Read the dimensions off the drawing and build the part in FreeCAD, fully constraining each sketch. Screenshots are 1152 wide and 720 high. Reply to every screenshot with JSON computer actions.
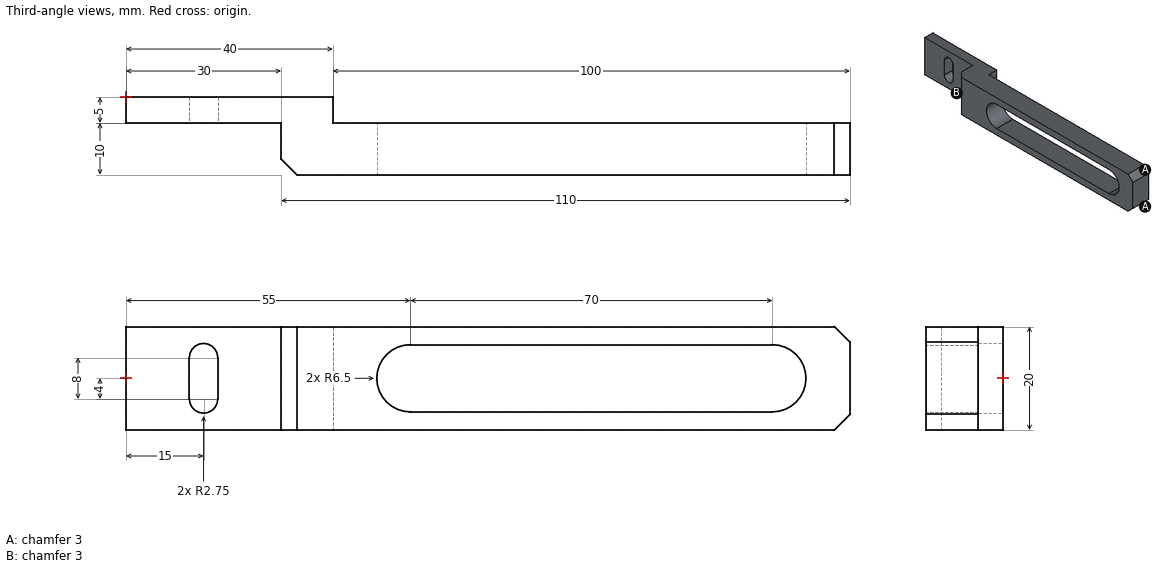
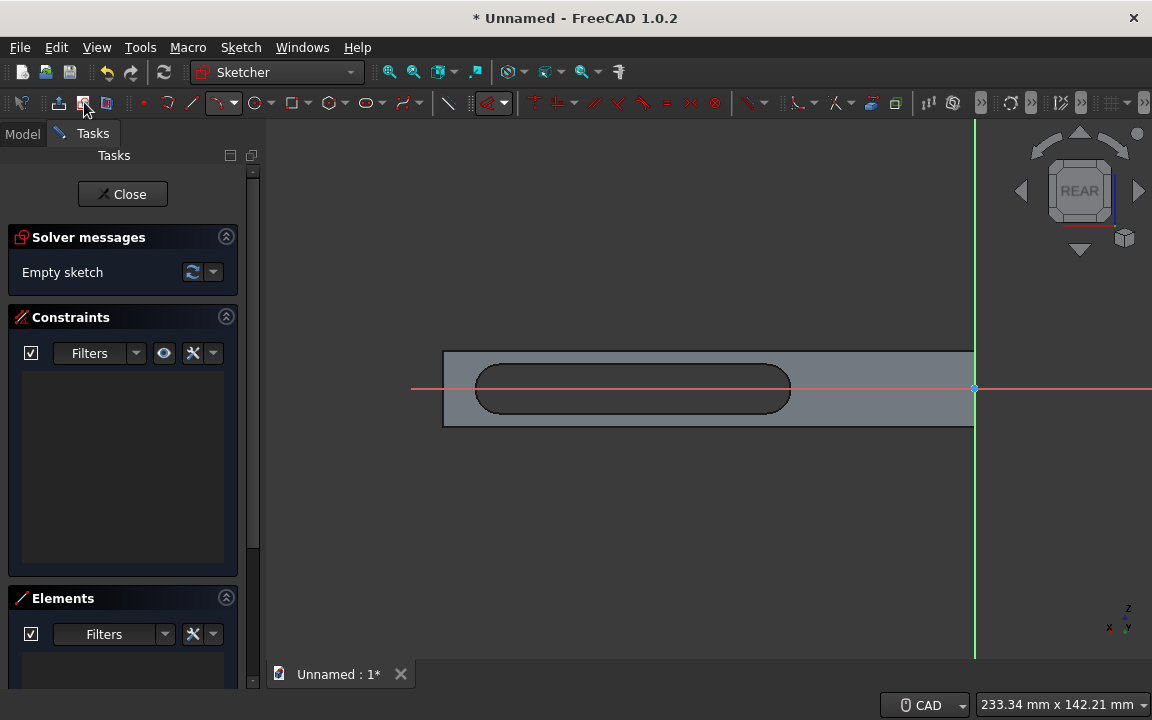
{"action": "scroll", "coordinate": [987, 389], "scroll_direction": "up", "scroll_amount": 9}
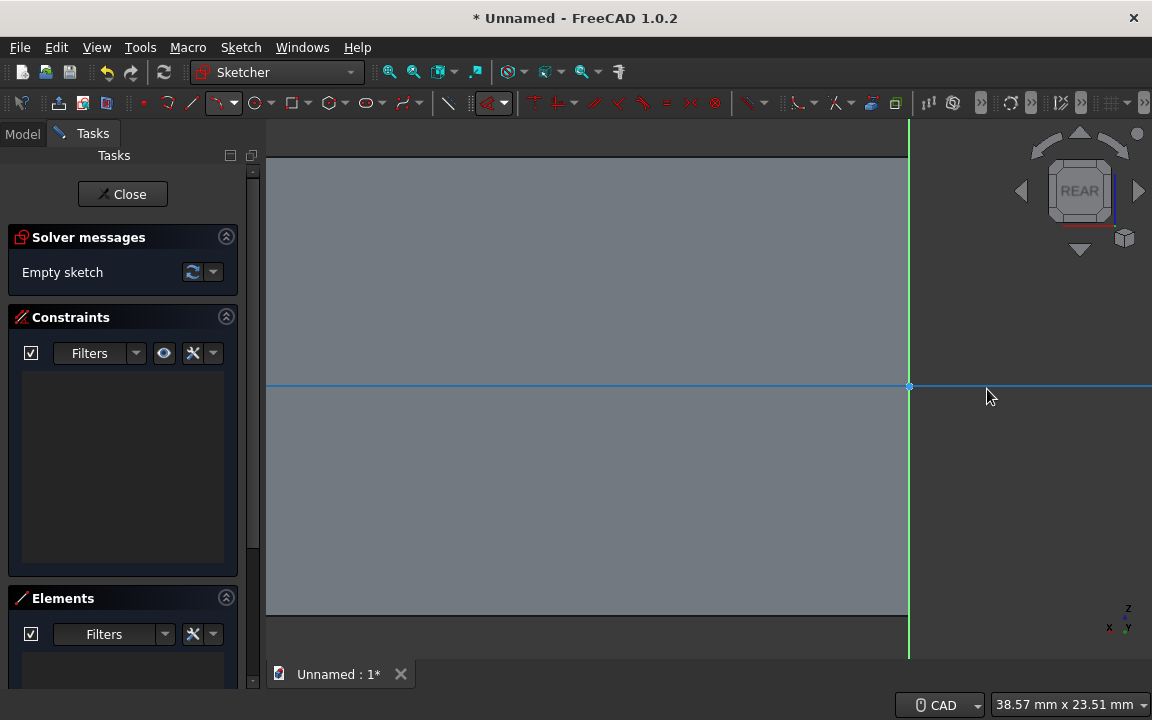
{"action": "left_click", "coordinate": [366, 104]}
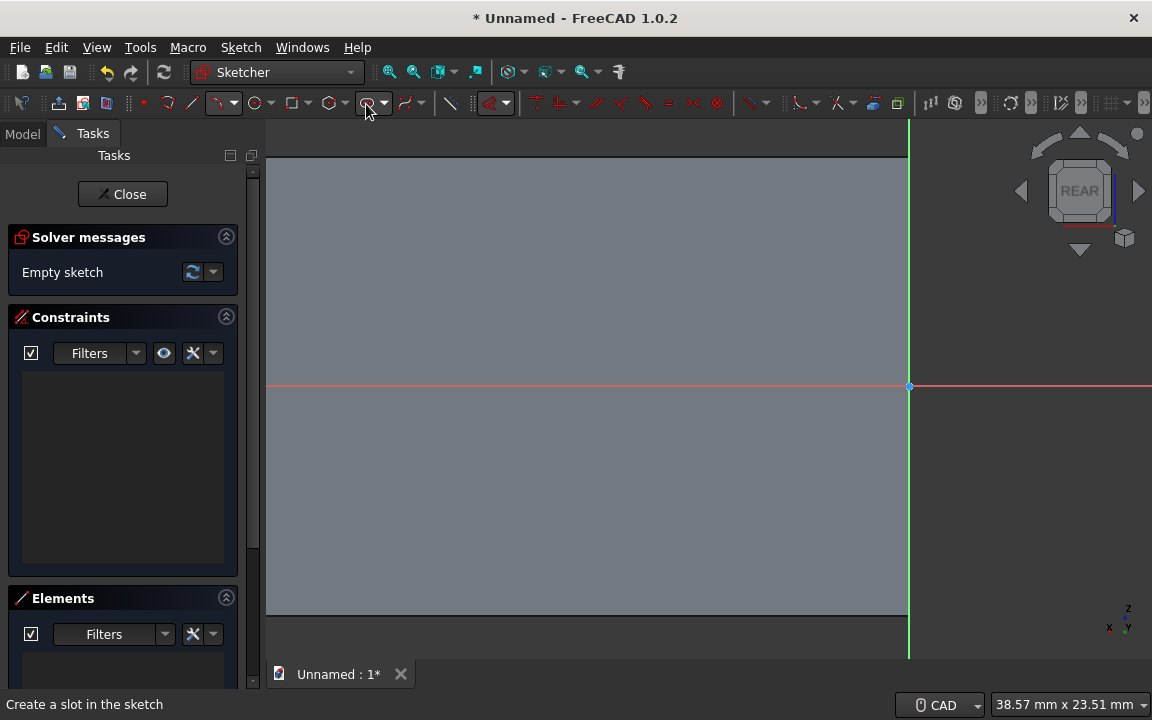
{"action": "left_click", "coordinate": [564, 478]}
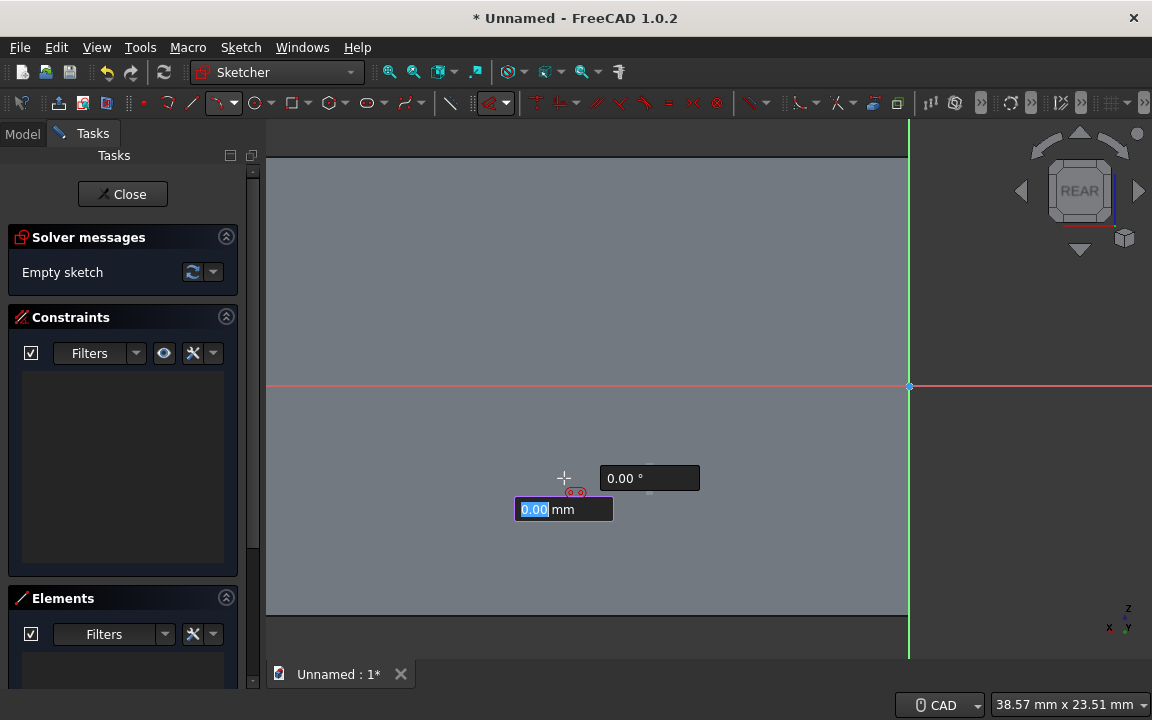
{"action": "left_click", "coordinate": [564, 295]}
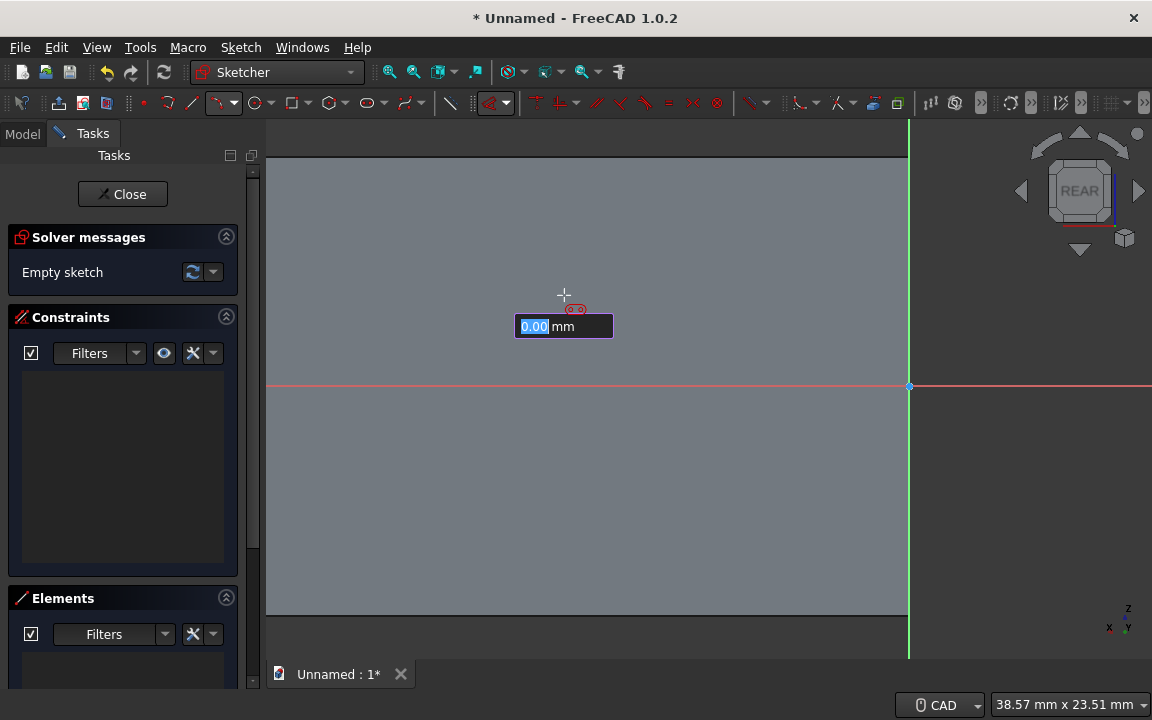
{"action": "left_click", "coordinate": [501, 359]}
{"action": "key", "text": "Escape"}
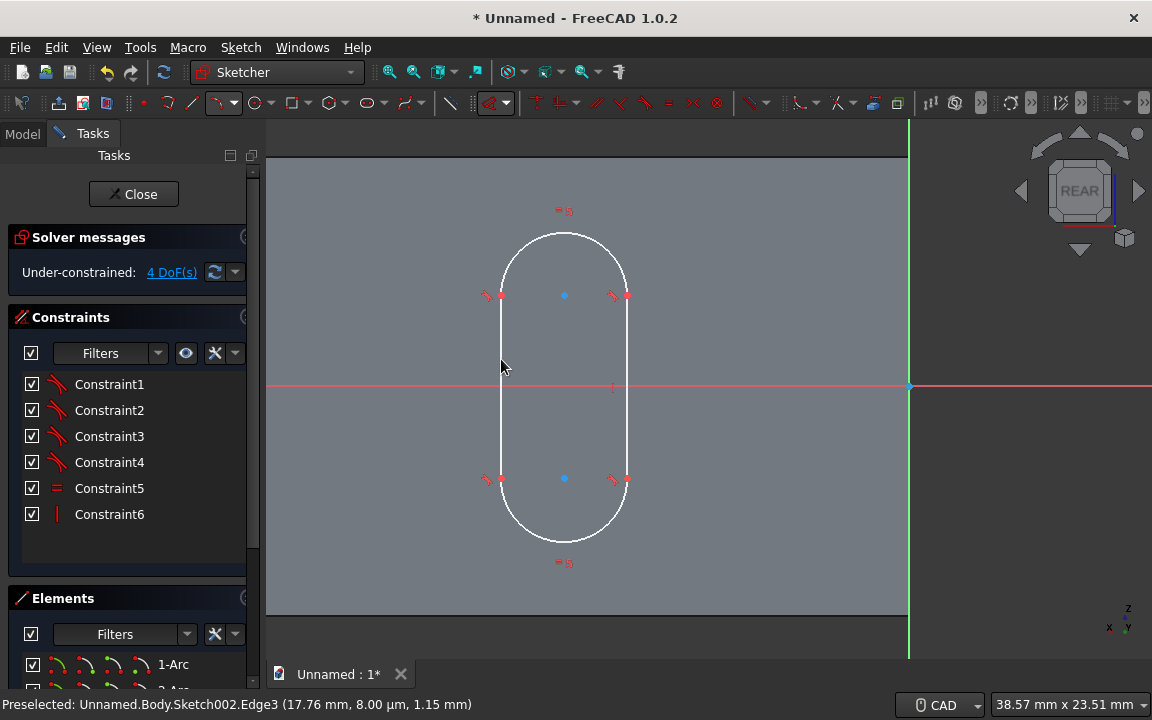
{"action": "left_click", "coordinate": [527, 530]}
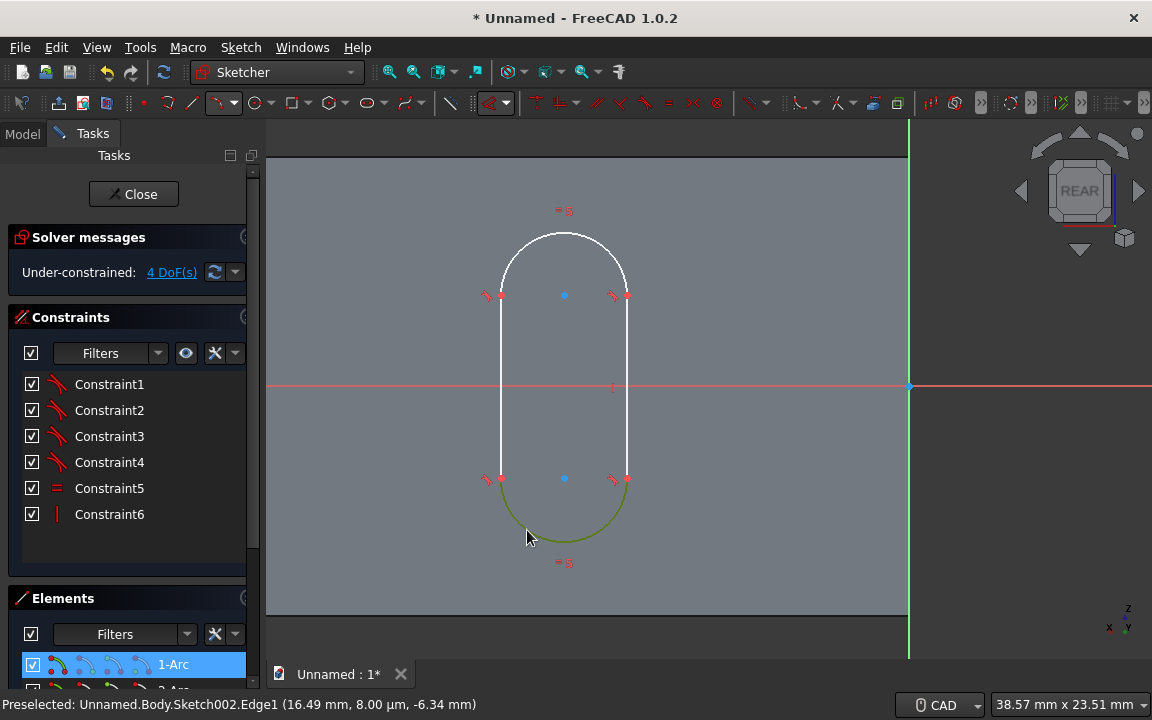
{"action": "key", "text": "k r"}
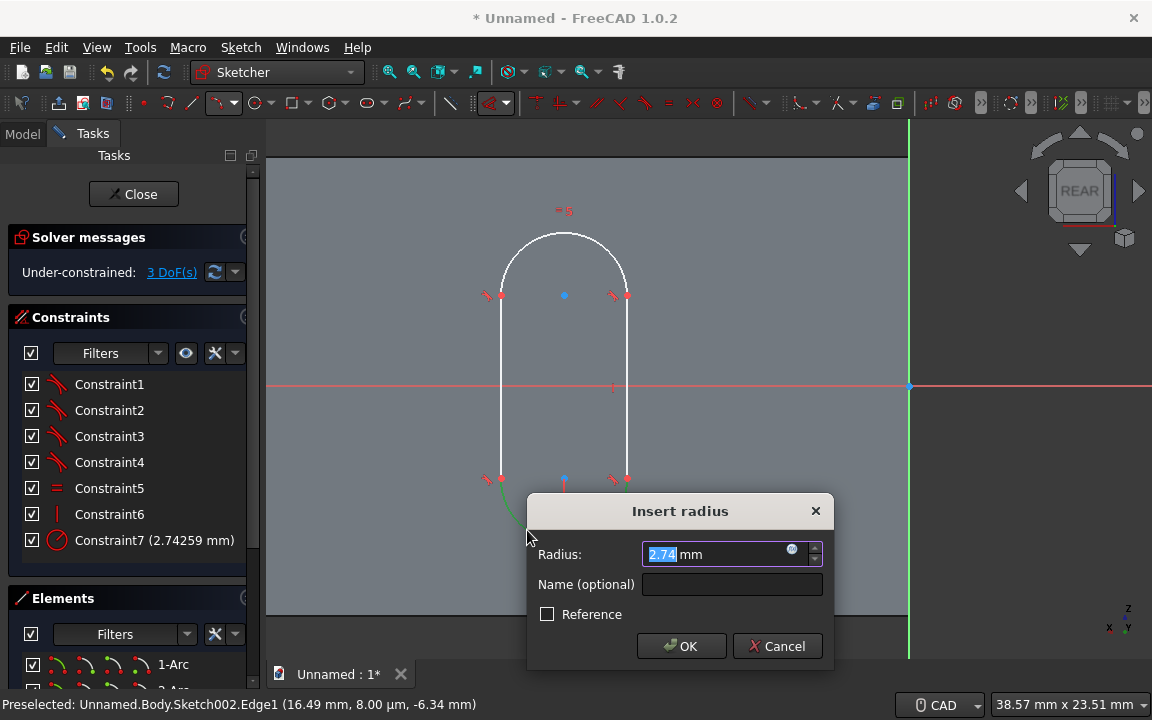
{"action": "type", "text": "2.75"}
{"action": "key", "text": "Return"}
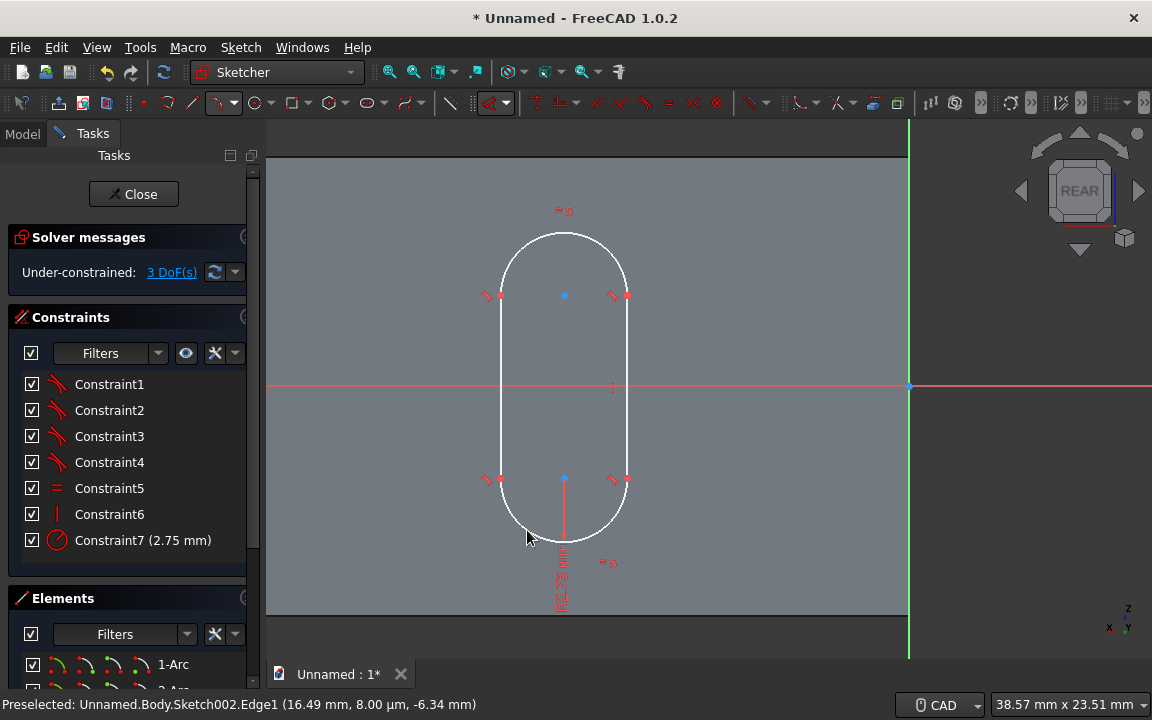
{"action": "left_click", "coordinate": [501, 424]}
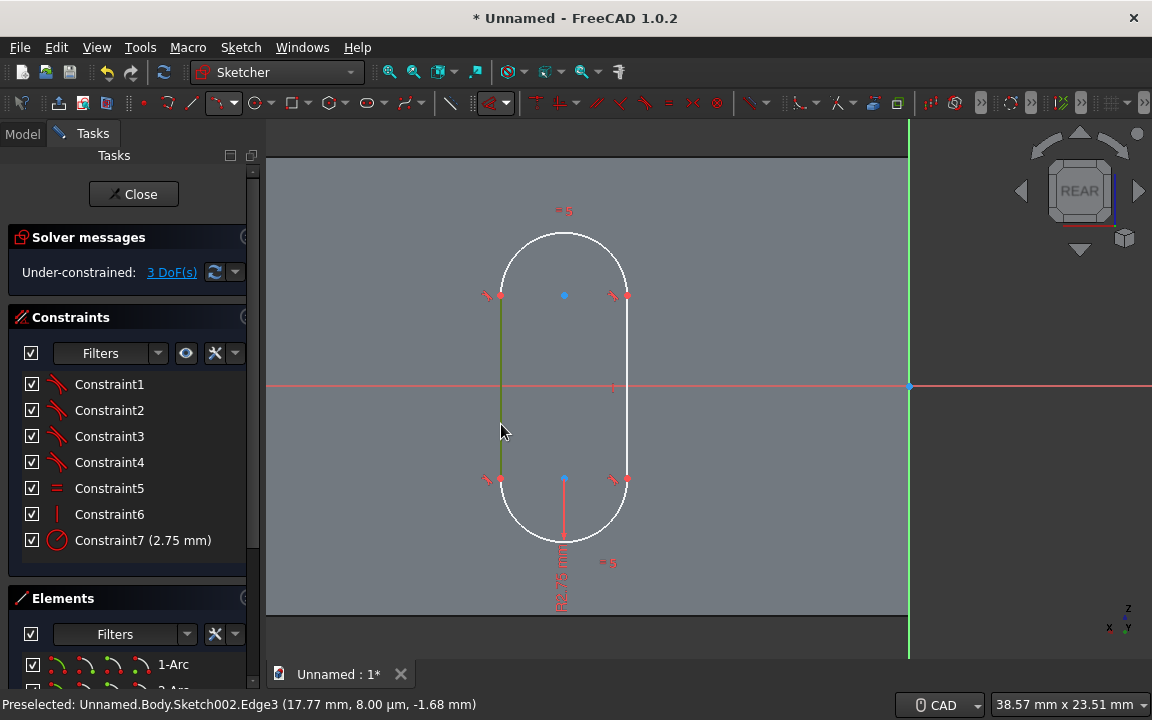
{"action": "key", "text": "i"}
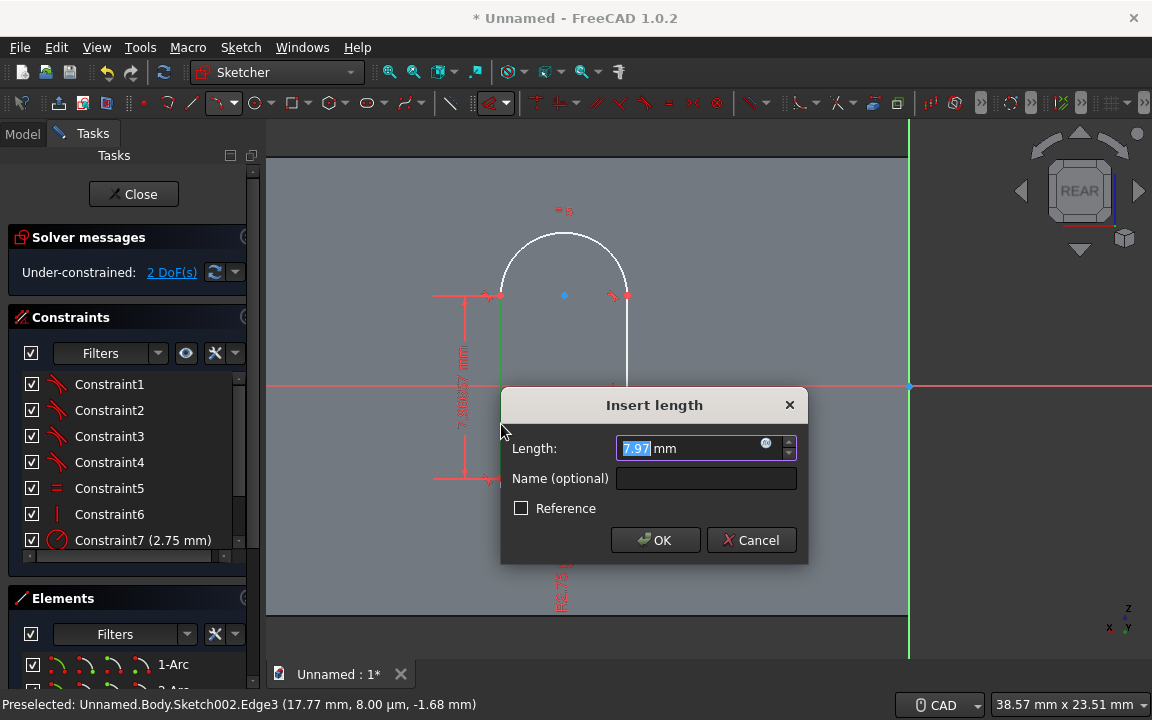
{"action": "type", "text": "8"}
{"action": "key", "text": "Return"}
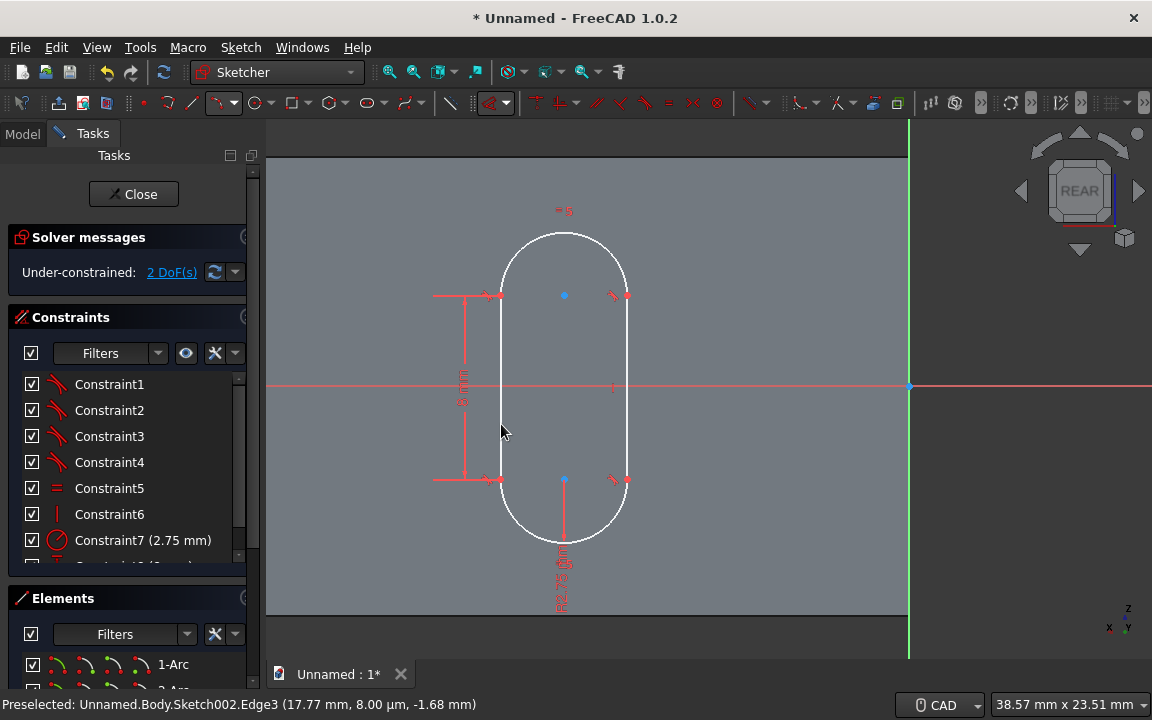
{"action": "left_click", "coordinate": [501, 480]}